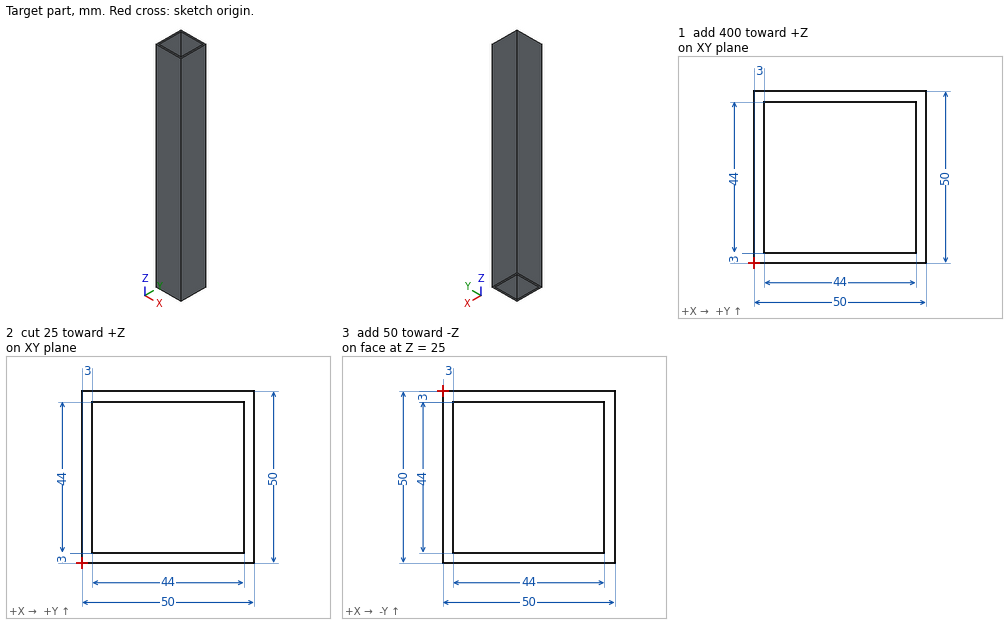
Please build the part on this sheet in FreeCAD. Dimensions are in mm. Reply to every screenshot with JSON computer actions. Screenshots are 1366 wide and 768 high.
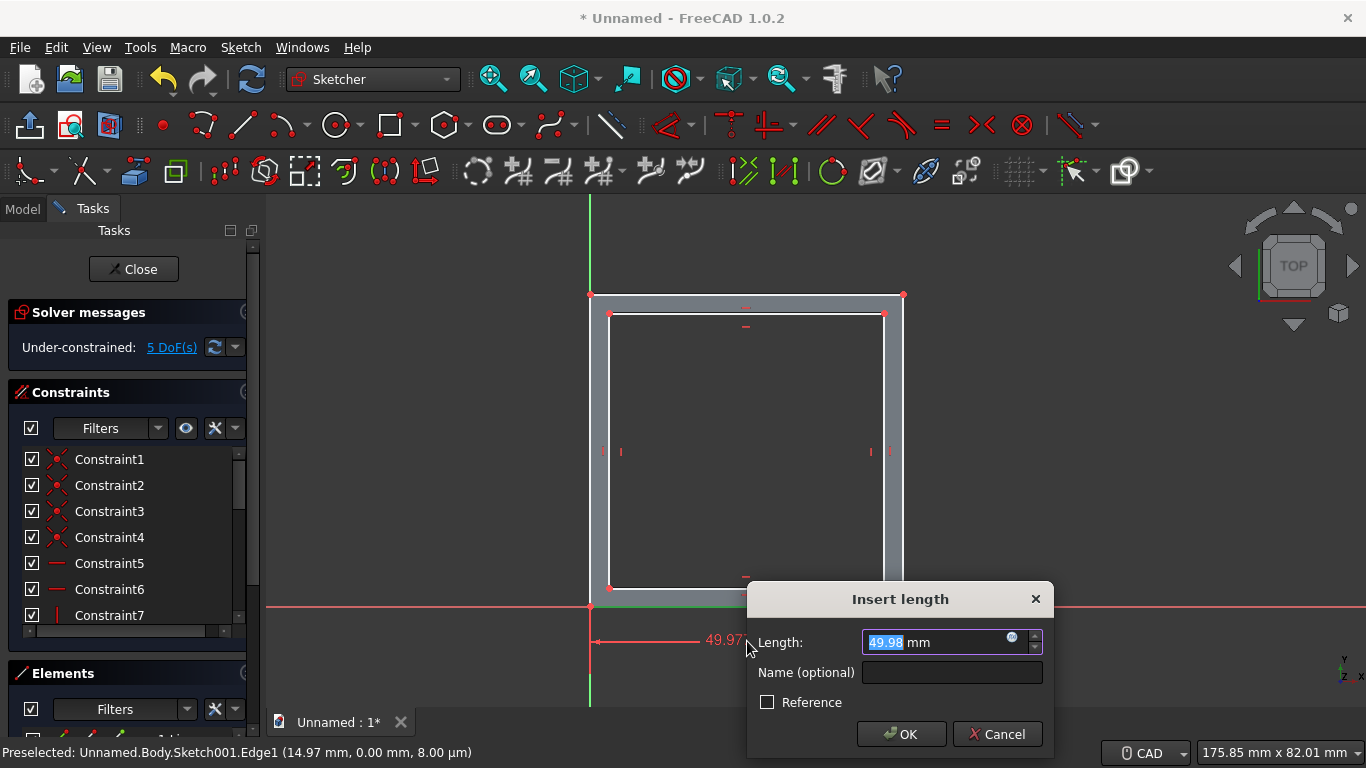
{"action": "type", "text": "50"}
{"action": "key", "text": "Return"}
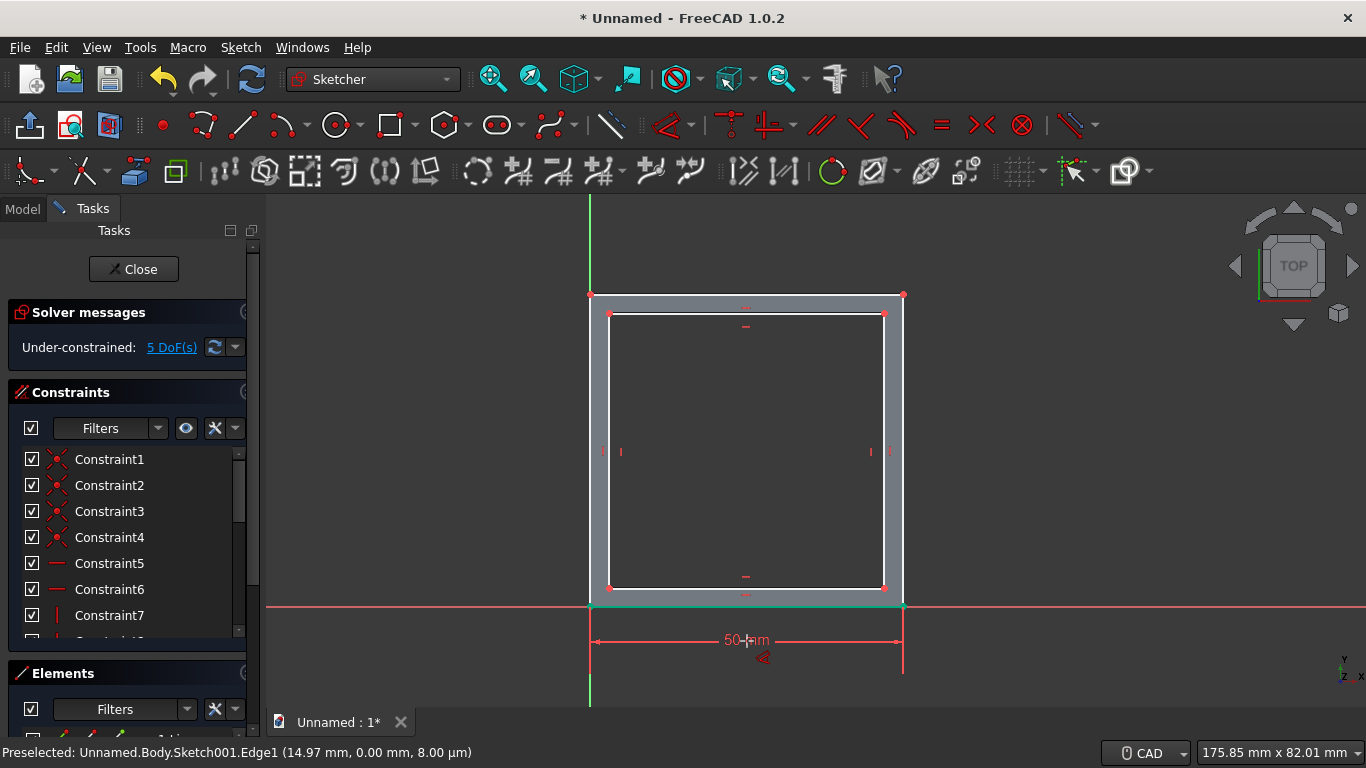
{"action": "left_click", "coordinate": [903, 513]}
{"action": "left_click", "coordinate": [937, 451]}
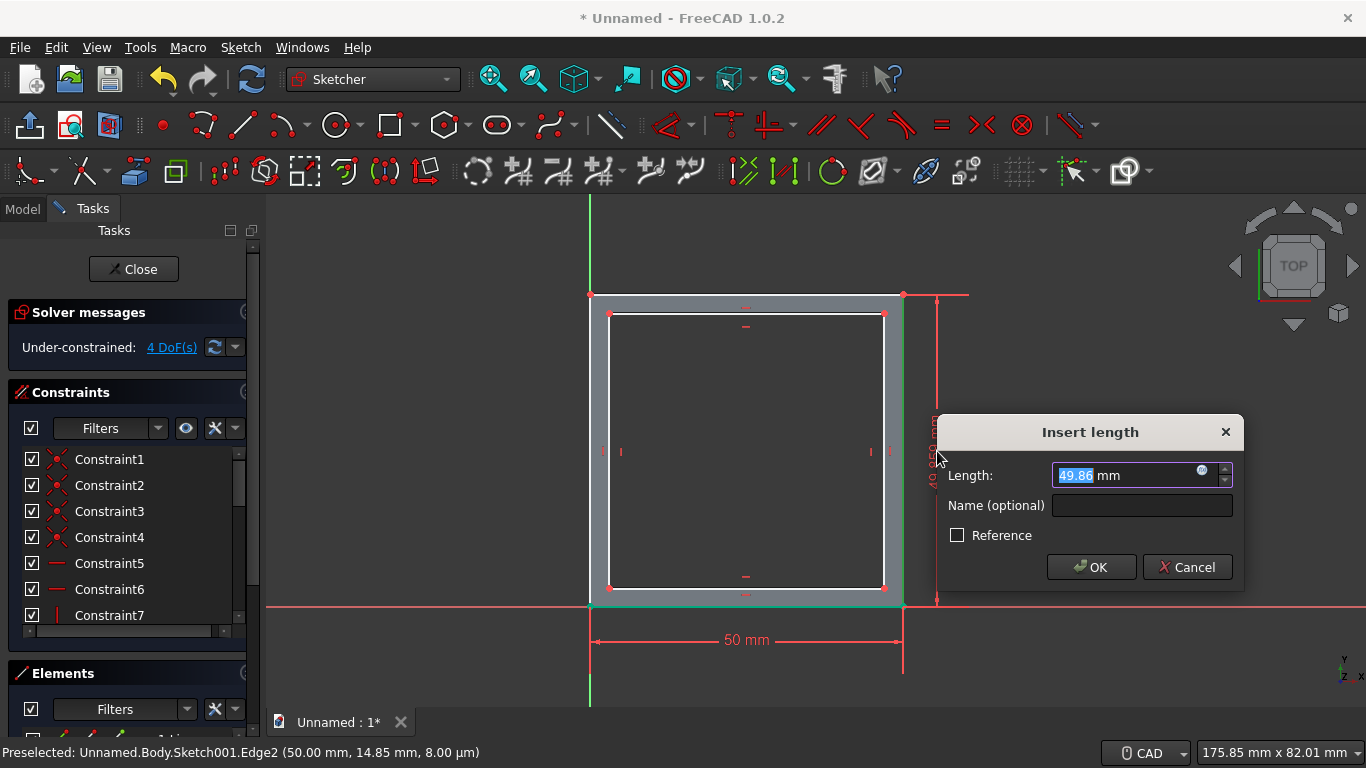
{"action": "type", "text": "50"}
{"action": "key", "text": "Return"}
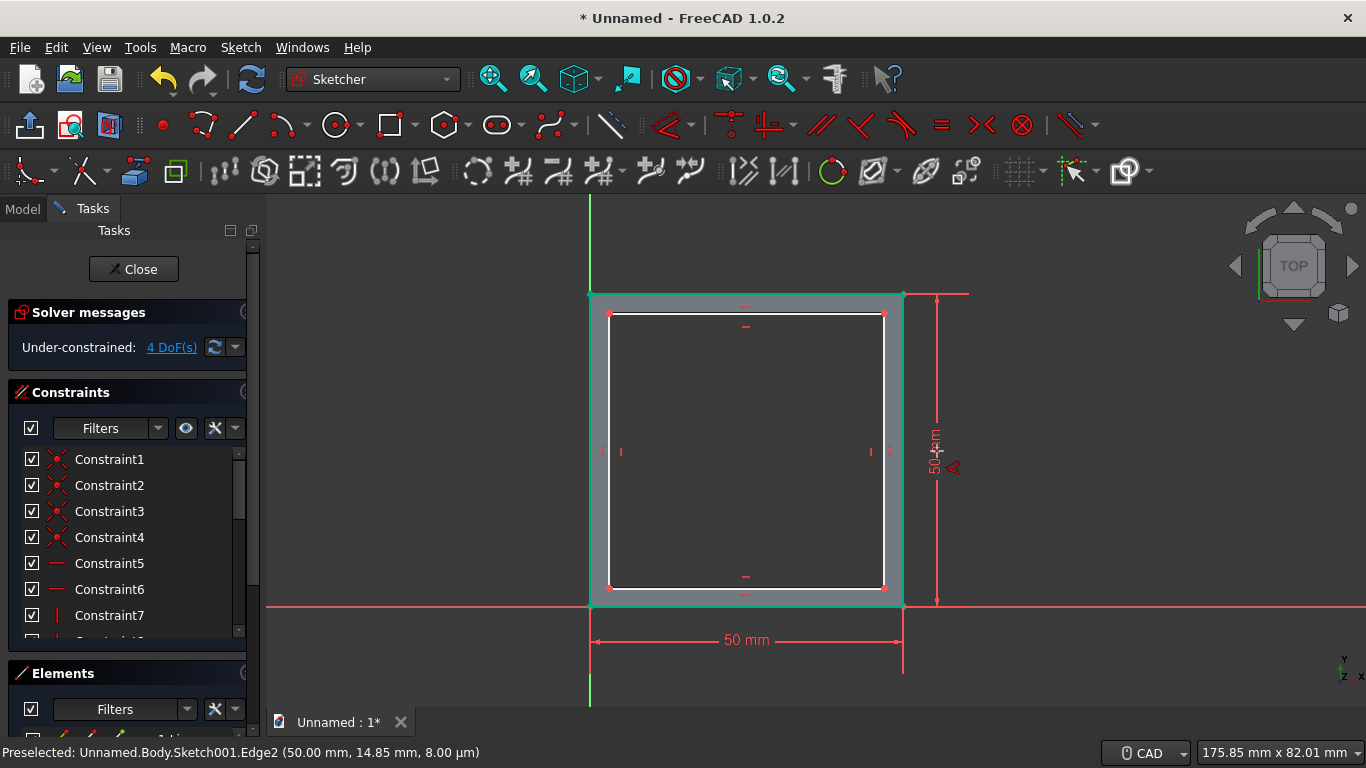
{"action": "left_click", "coordinate": [609, 396]}
{"action": "left_click", "coordinate": [575, 451]}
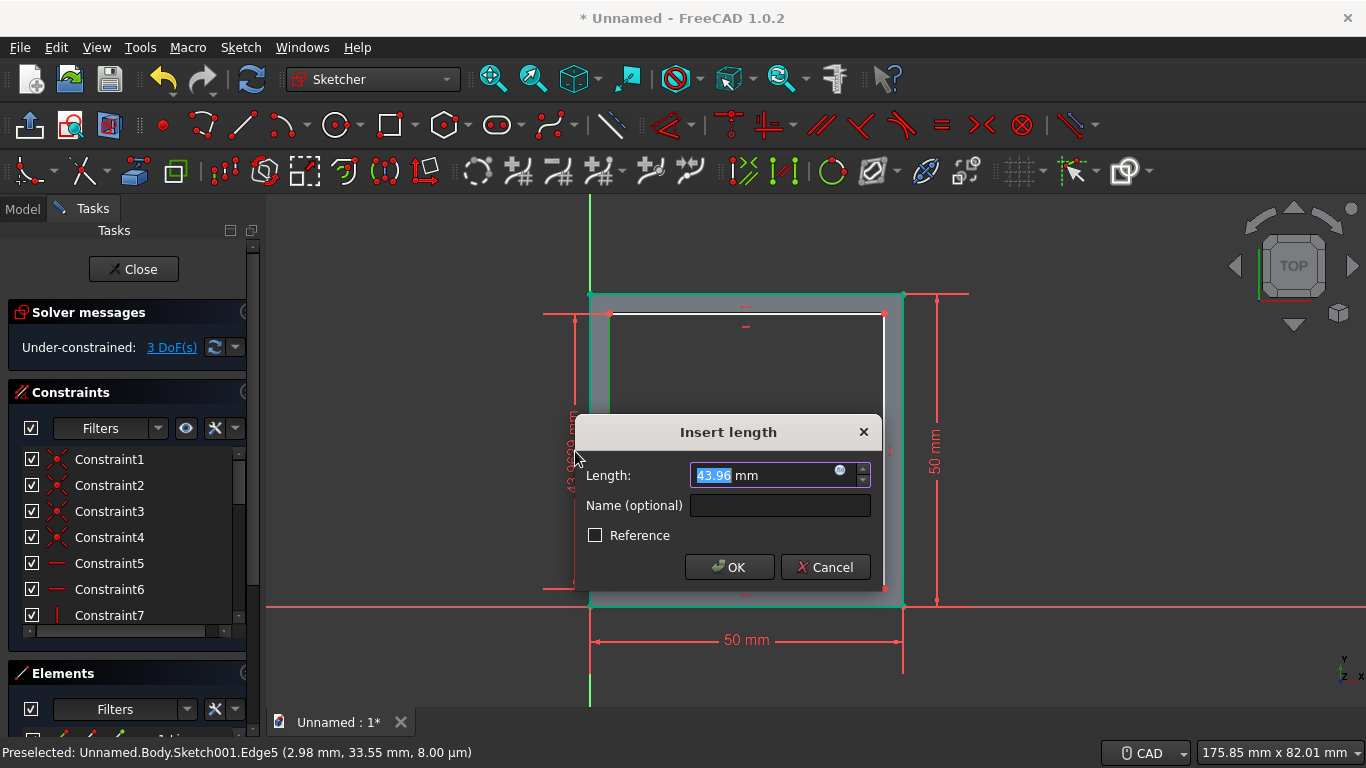
{"action": "type", "text": "44"}
{"action": "key", "text": "Return"}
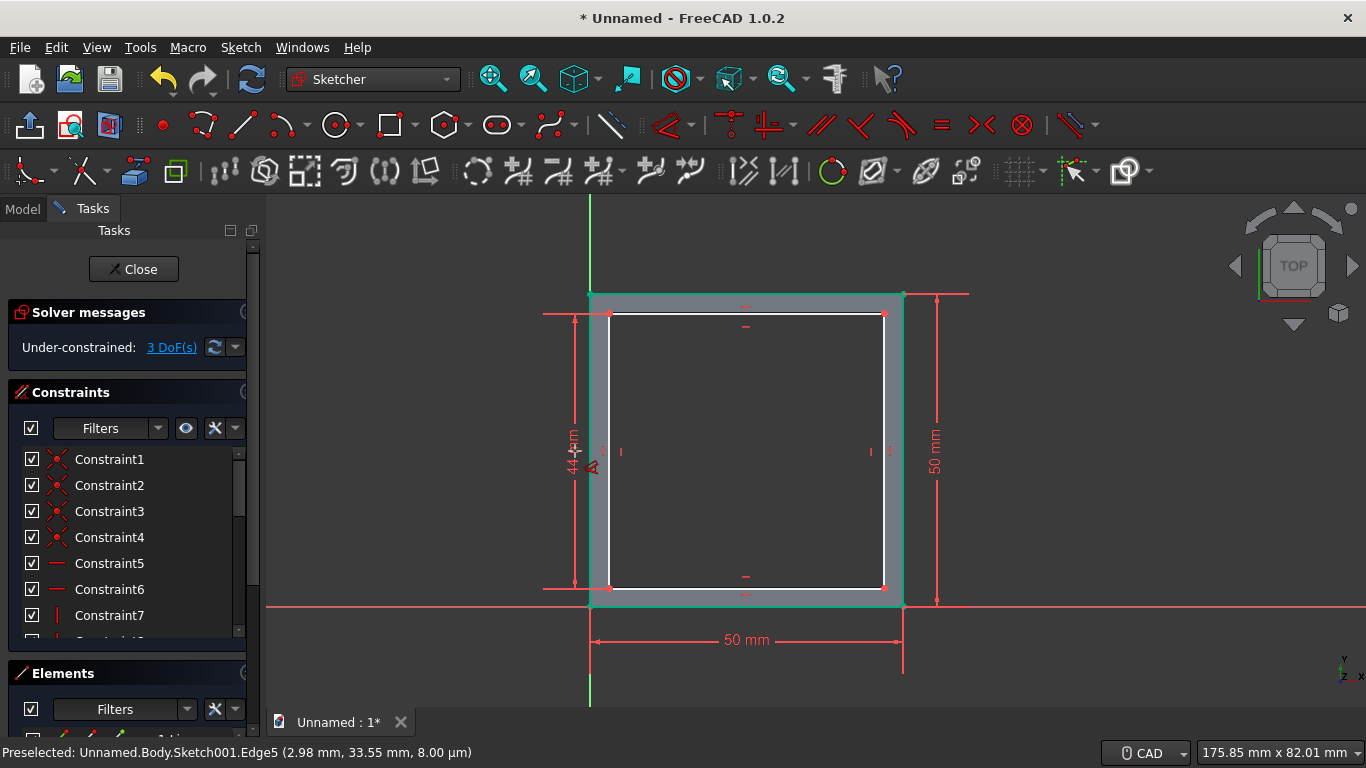
{"action": "left_click", "coordinate": [692, 589]}
{"action": "left_click", "coordinate": [650, 623]}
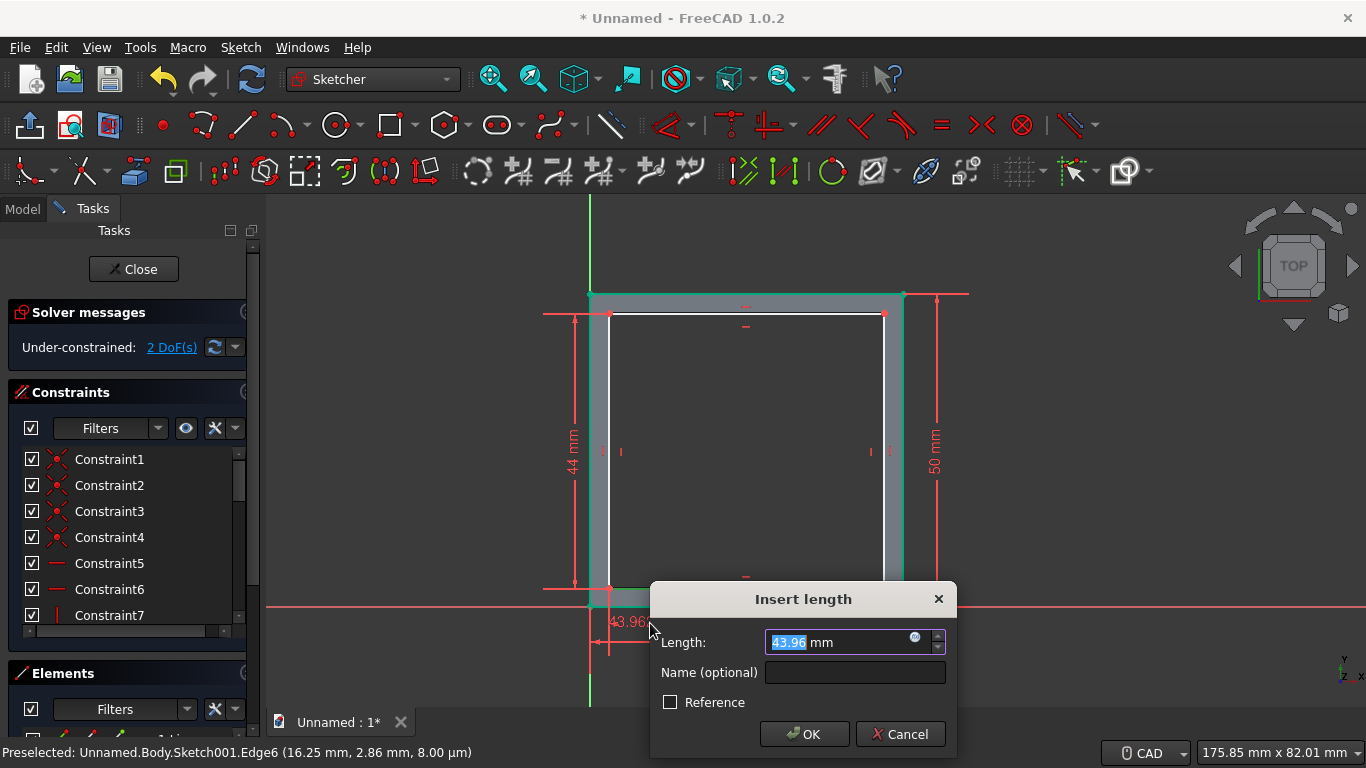
{"action": "type", "text": "44"}
{"action": "key", "text": "Return"}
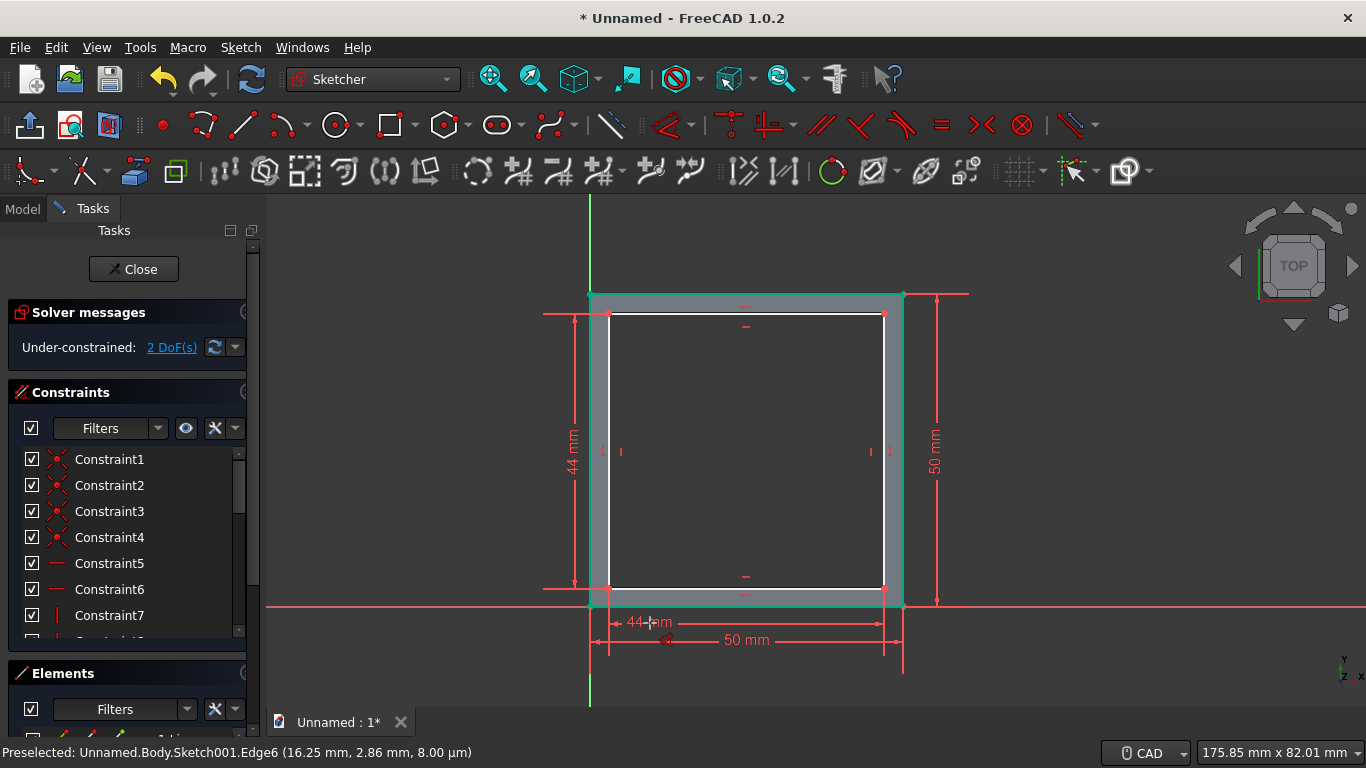
{"action": "scroll", "coordinate": [609, 314], "scroll_direction": "up", "scroll_amount": 4}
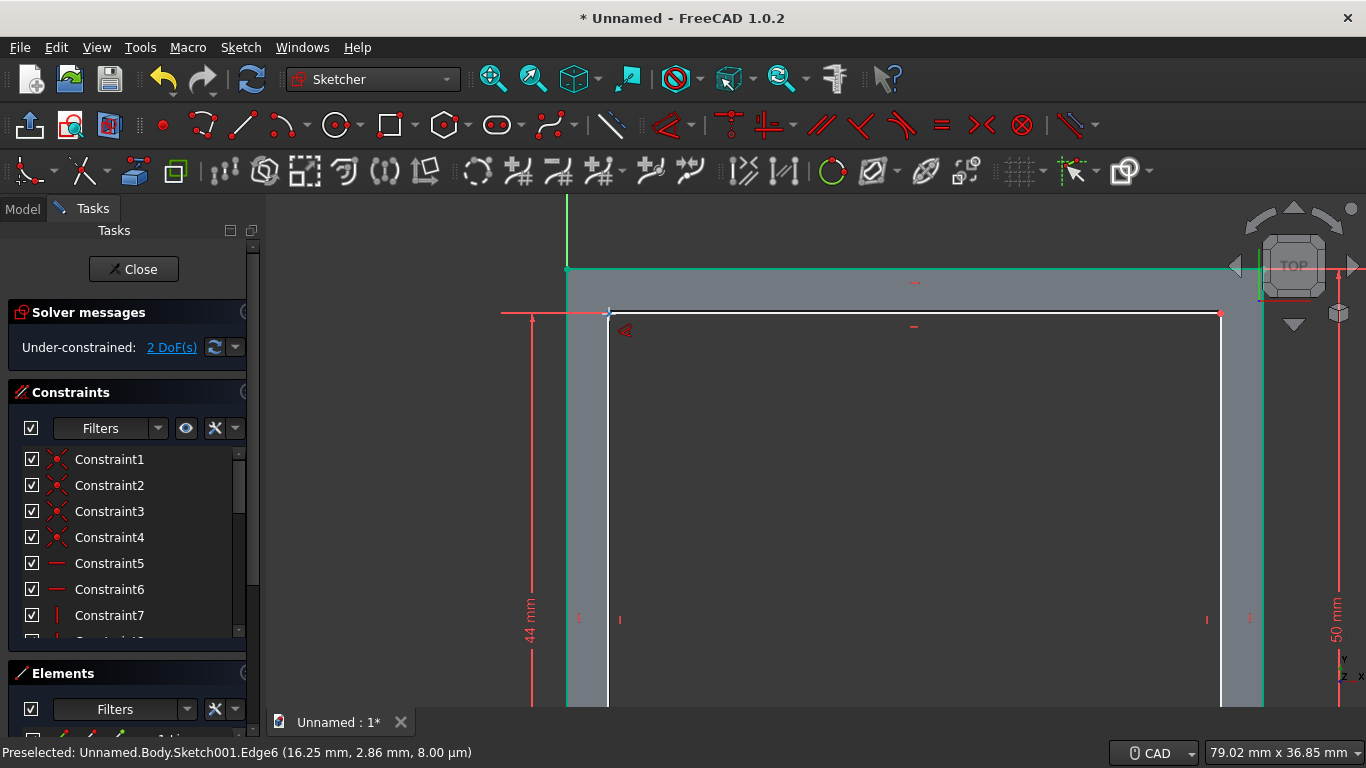
{"action": "left_click", "coordinate": [608, 313]}
{"action": "left_click", "coordinate": [588, 255]}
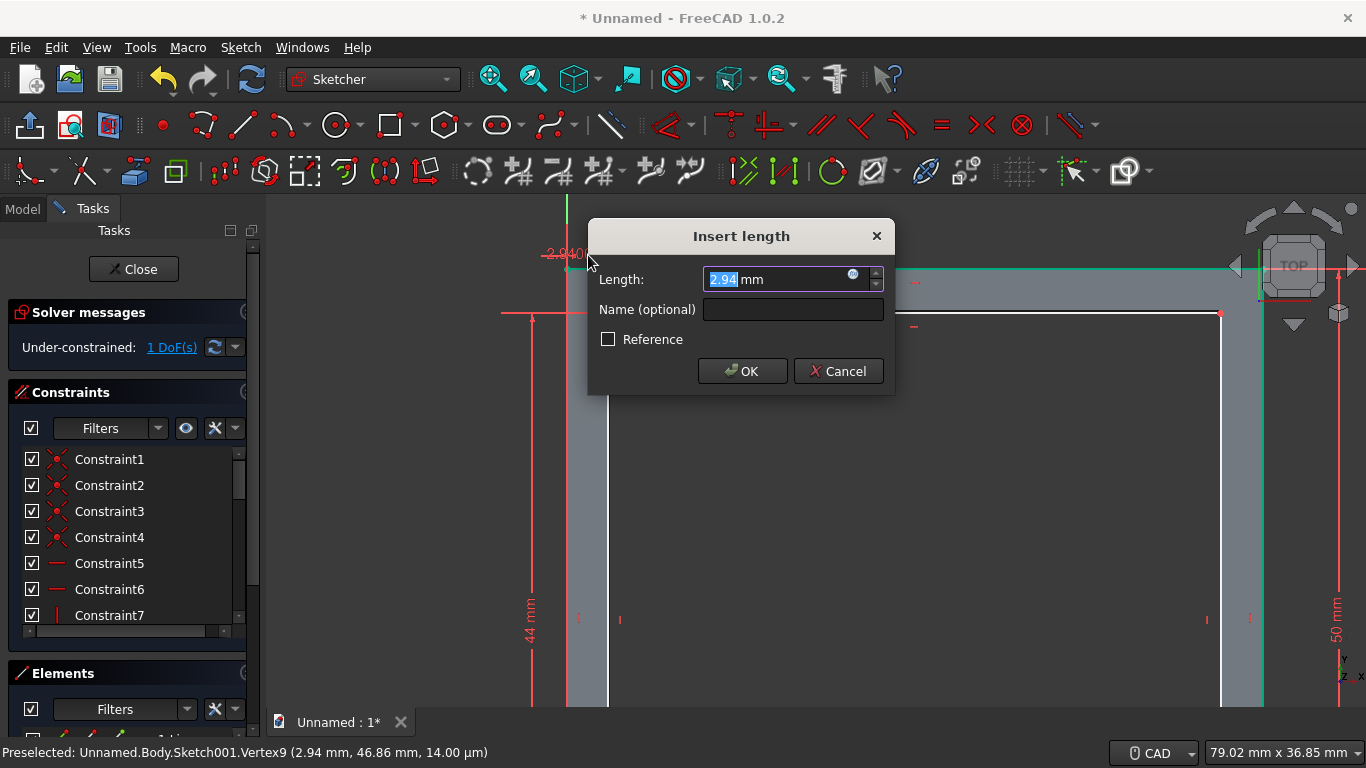
{"action": "type", "text": "3"}
{"action": "key", "text": "Return"}